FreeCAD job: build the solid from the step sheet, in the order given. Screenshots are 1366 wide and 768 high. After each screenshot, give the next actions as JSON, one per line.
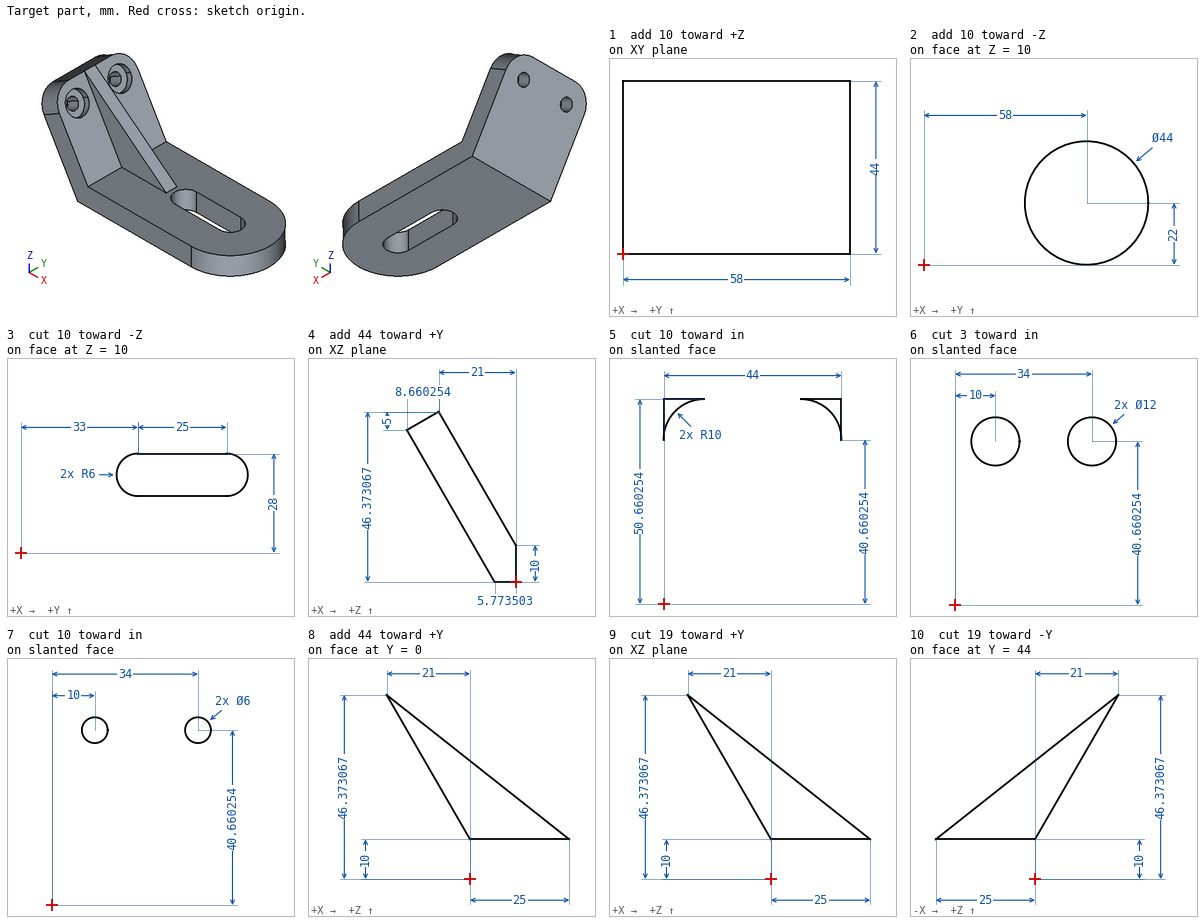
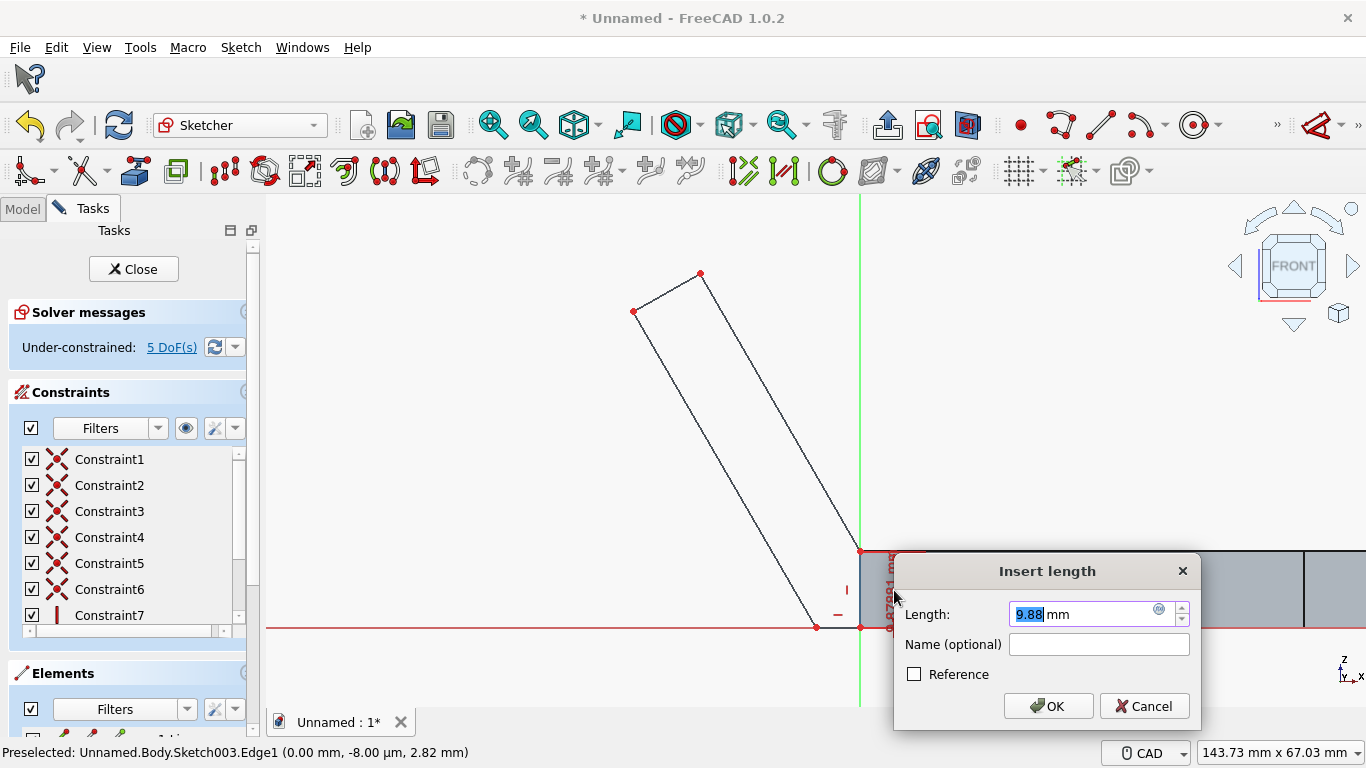
{"action": "type", "text": "10"}
{"action": "key", "text": "Return"}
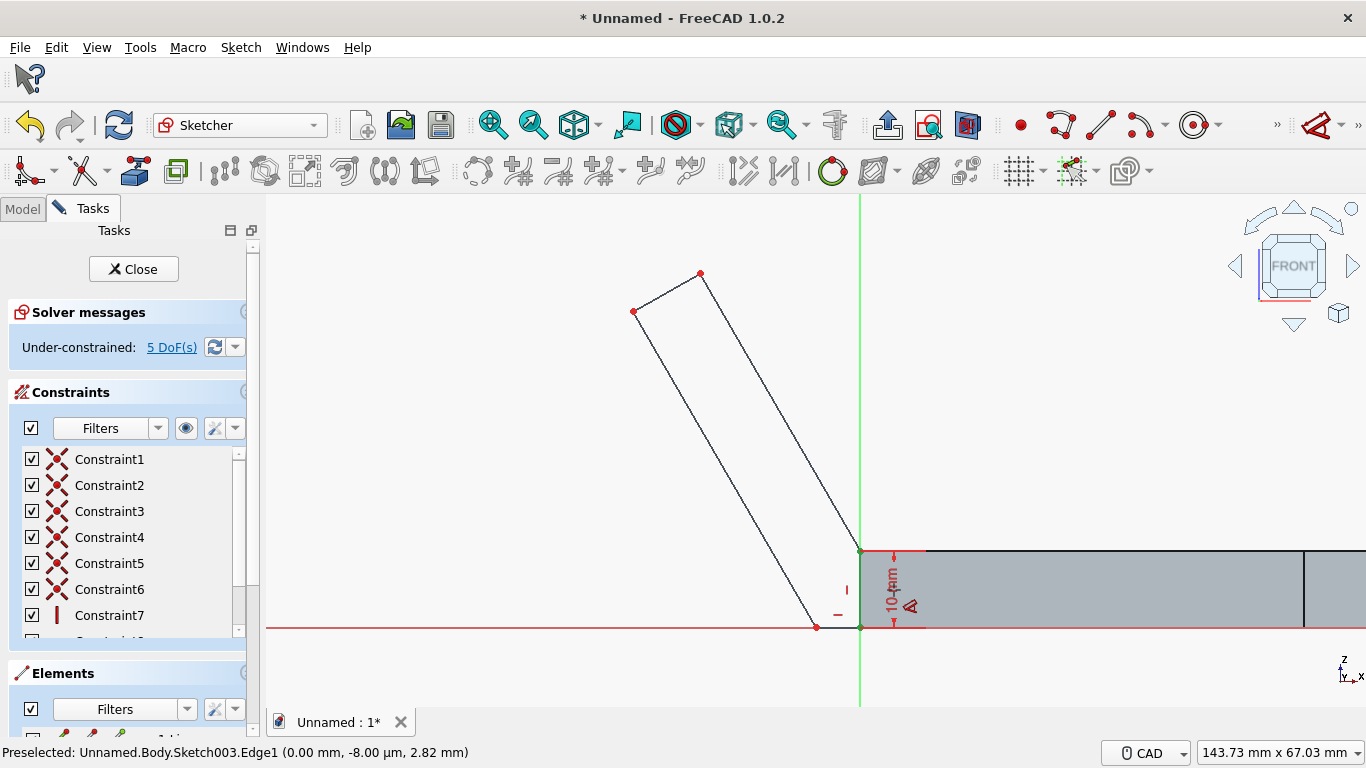
{"action": "left_click", "coordinate": [680, 285]}
{"action": "left_click", "coordinate": [599, 293]}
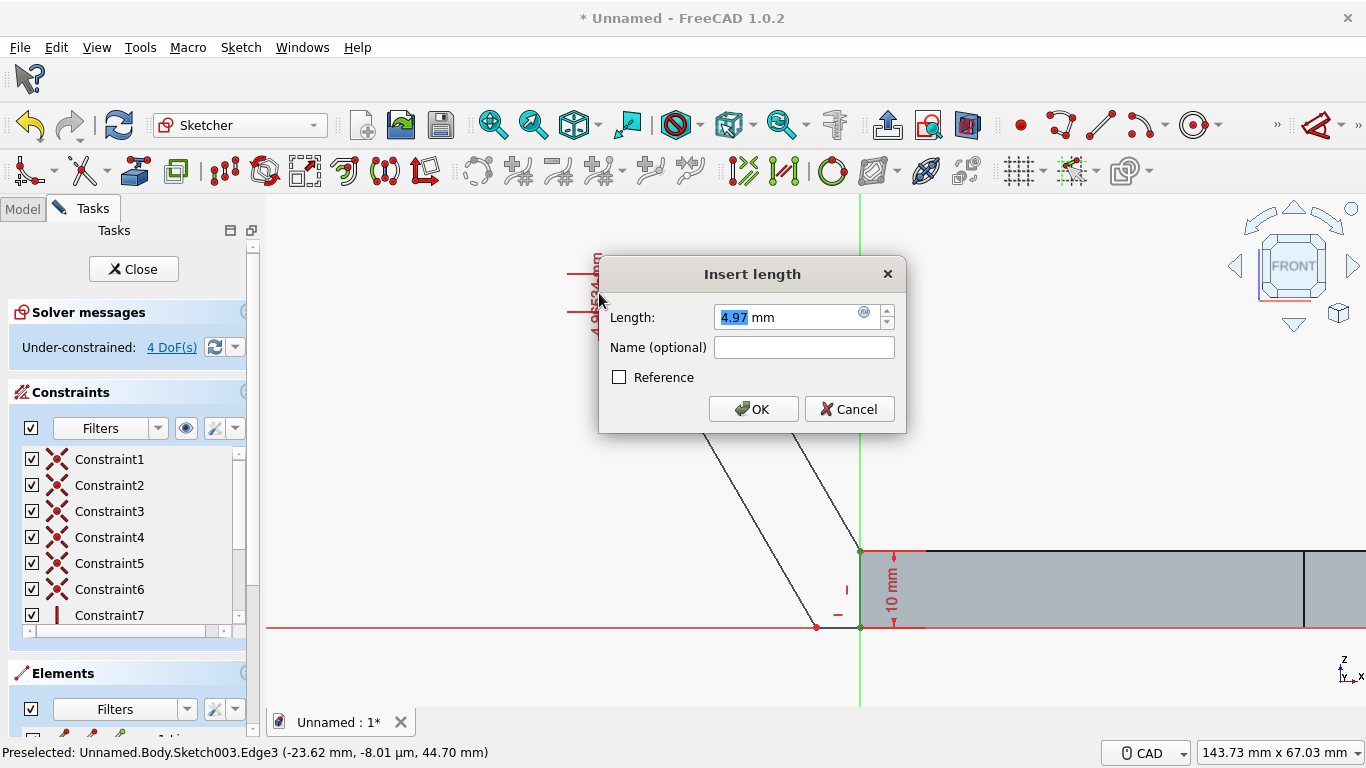
{"action": "type", "text": "5"}
{"action": "key", "text": "Return"}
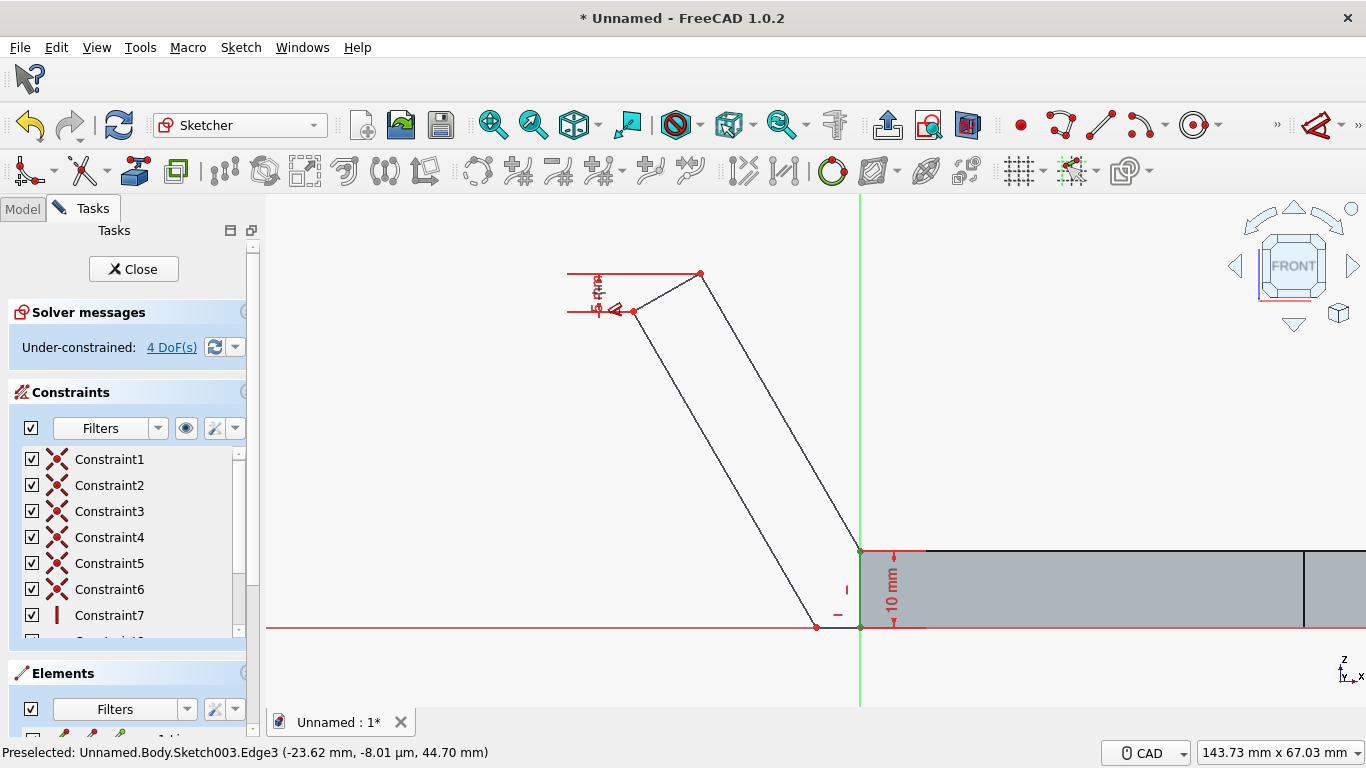
{"action": "left_click", "coordinate": [700, 274]}
{"action": "left_click", "coordinate": [780, 662]}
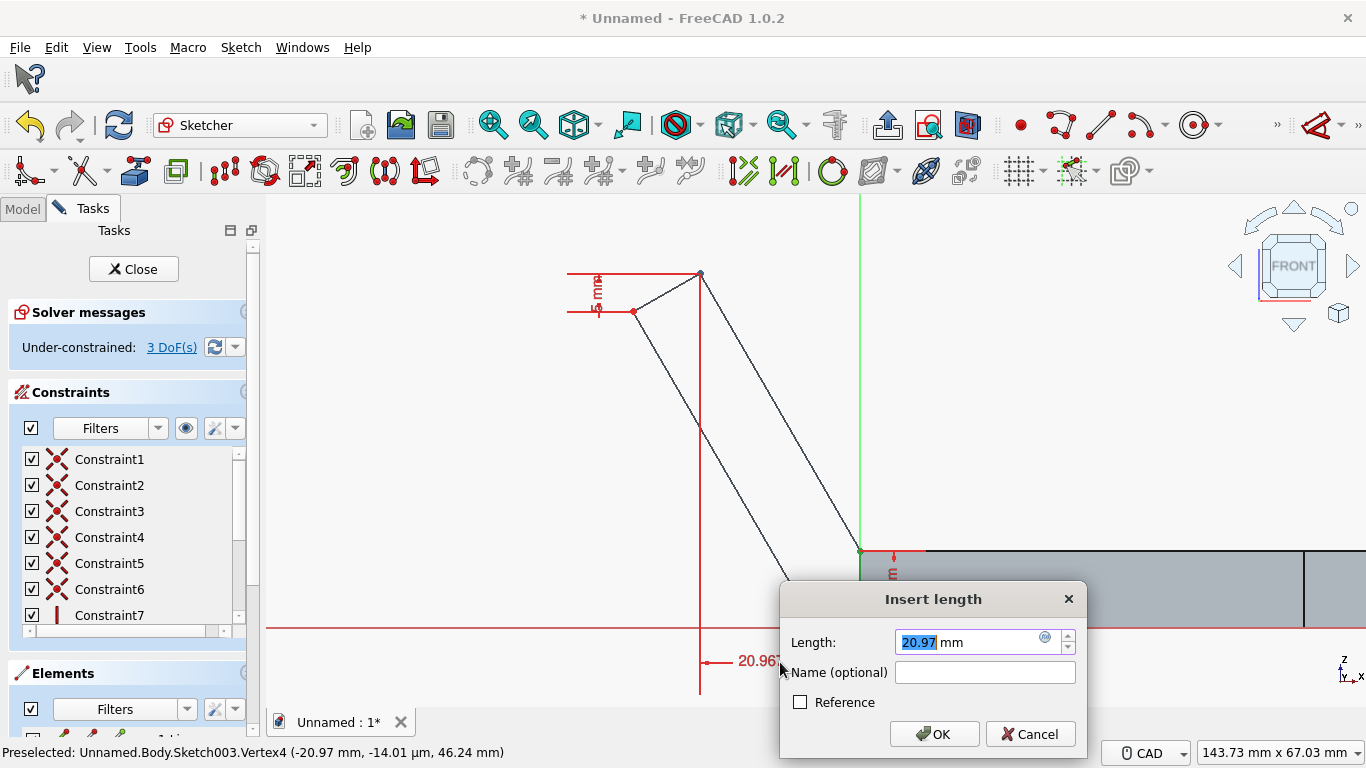
{"action": "type", "text": "21"}
{"action": "key", "text": "Return"}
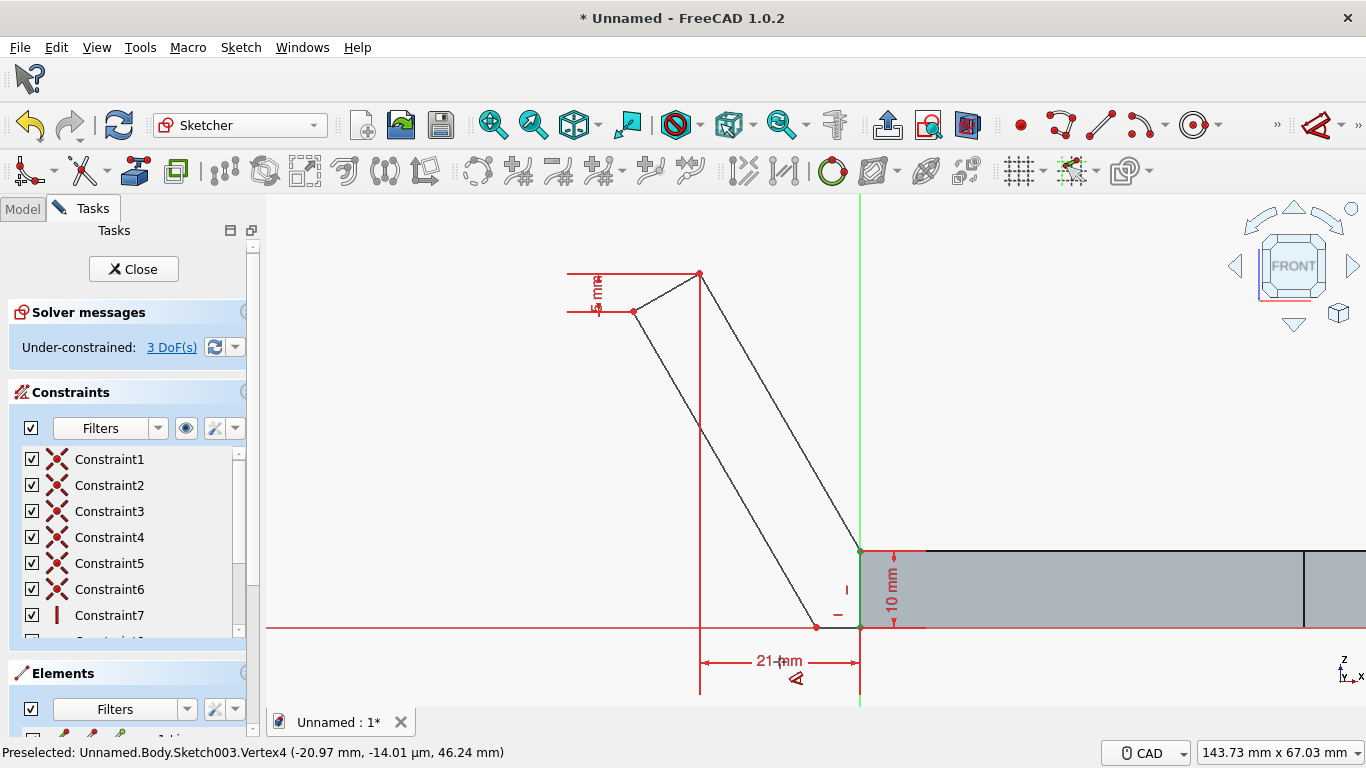
{"action": "left_click", "coordinate": [829, 628]}
{"action": "left_click", "coordinate": [823, 594]}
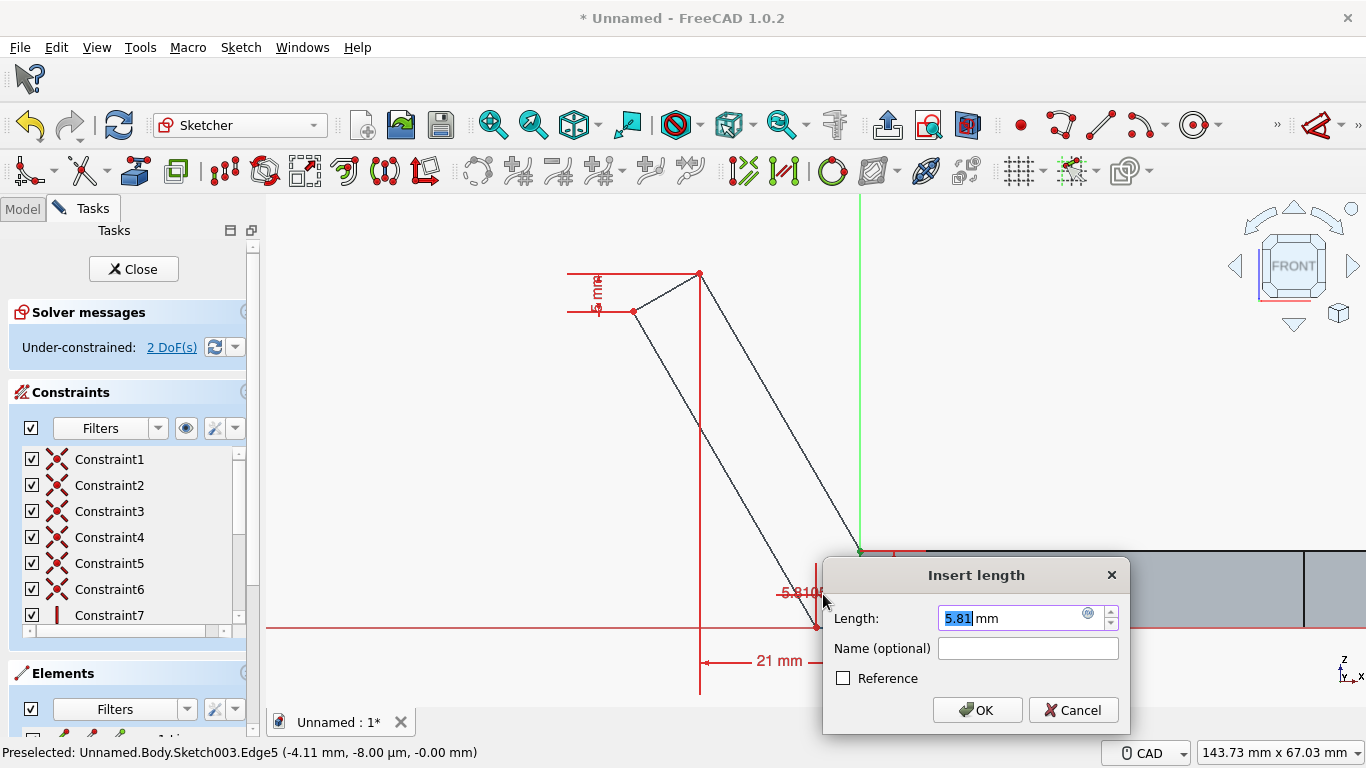
{"action": "type", "text": "5.773503"}
{"action": "key", "text": "Return"}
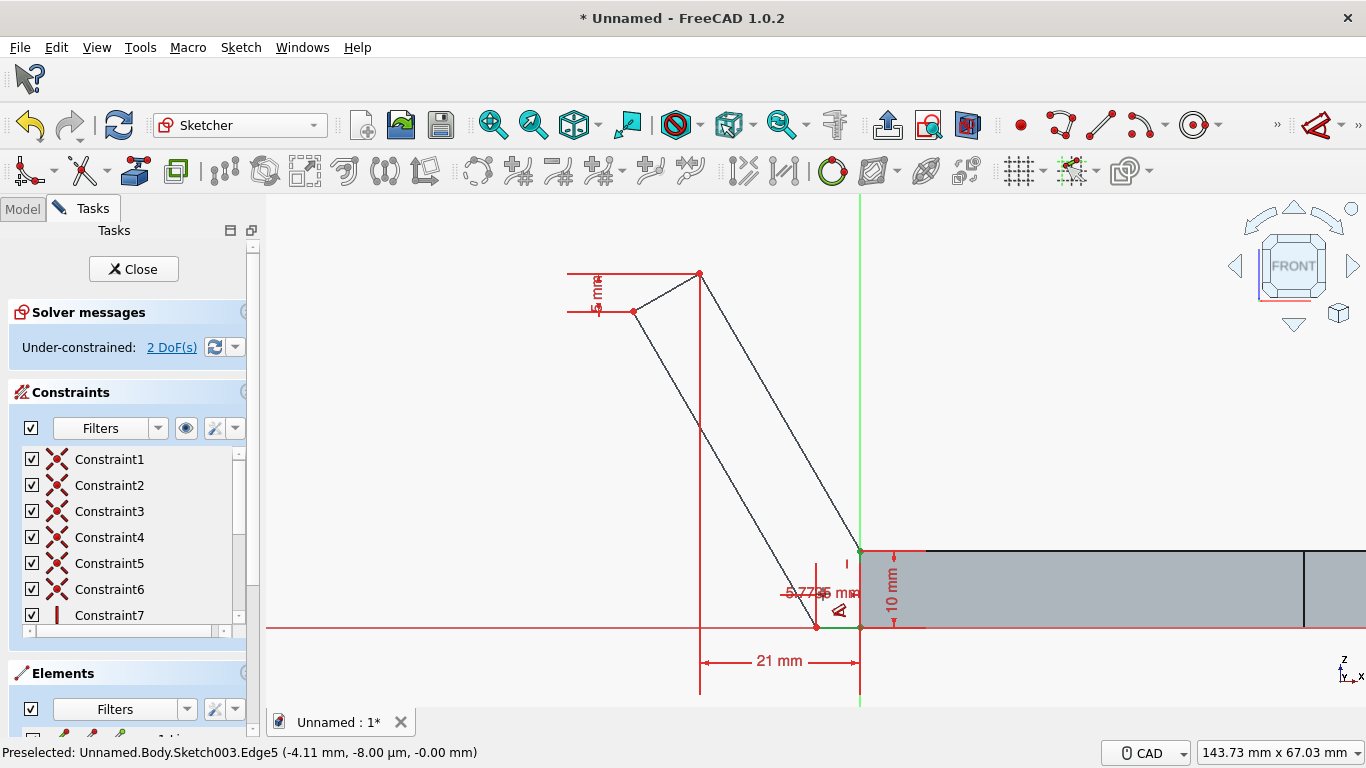
{"action": "left_click", "coordinate": [680, 285]}
{"action": "left_click", "coordinate": [666, 240]}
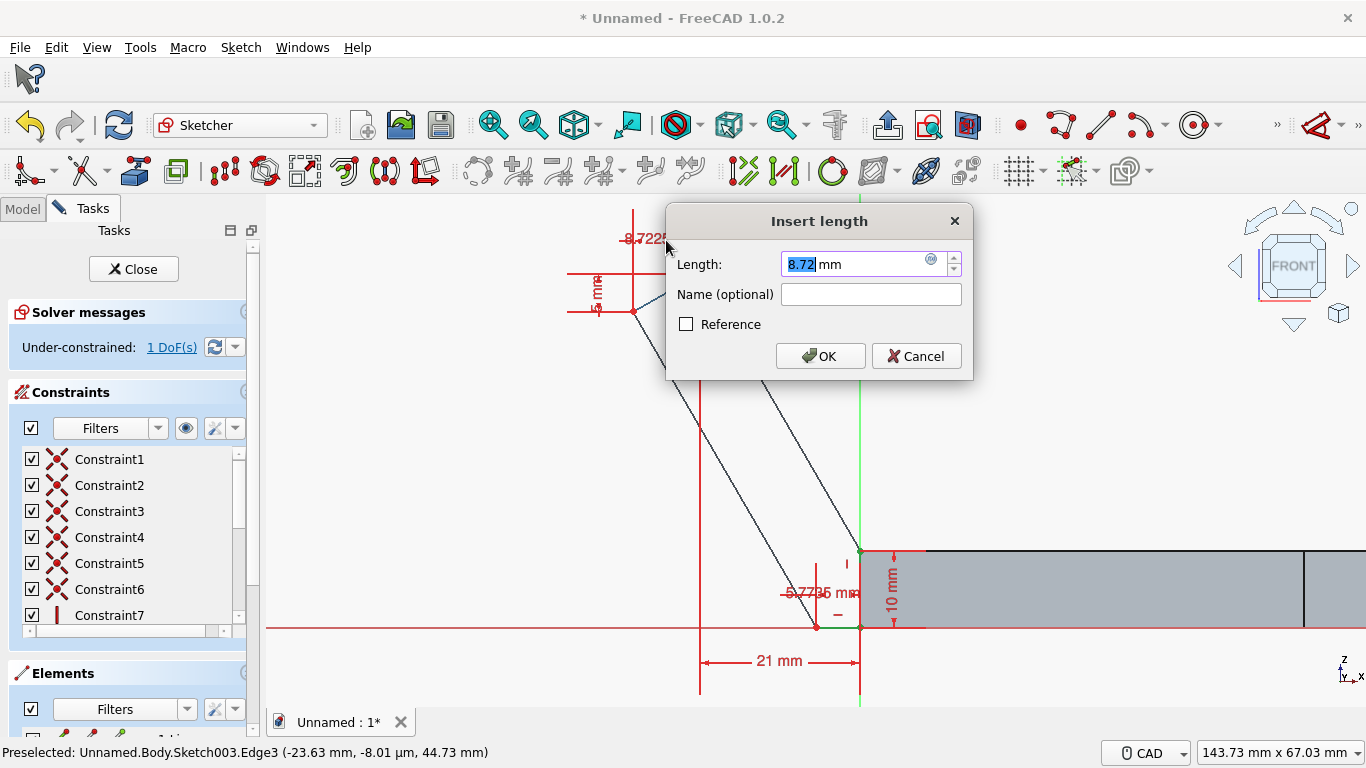
{"action": "type", "text": "8.660254"}
{"action": "key", "text": "Return"}